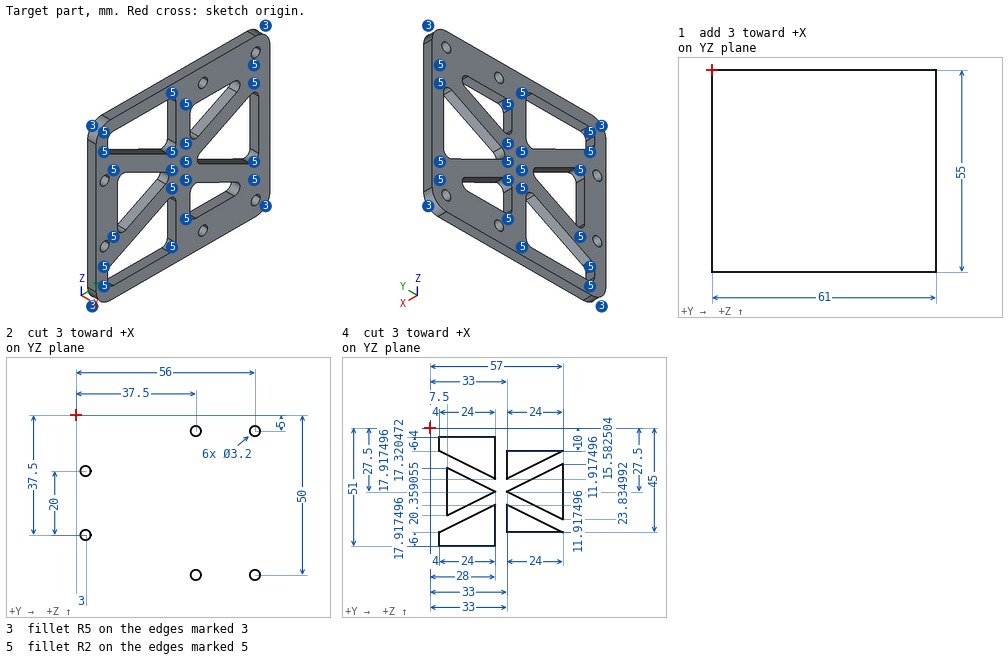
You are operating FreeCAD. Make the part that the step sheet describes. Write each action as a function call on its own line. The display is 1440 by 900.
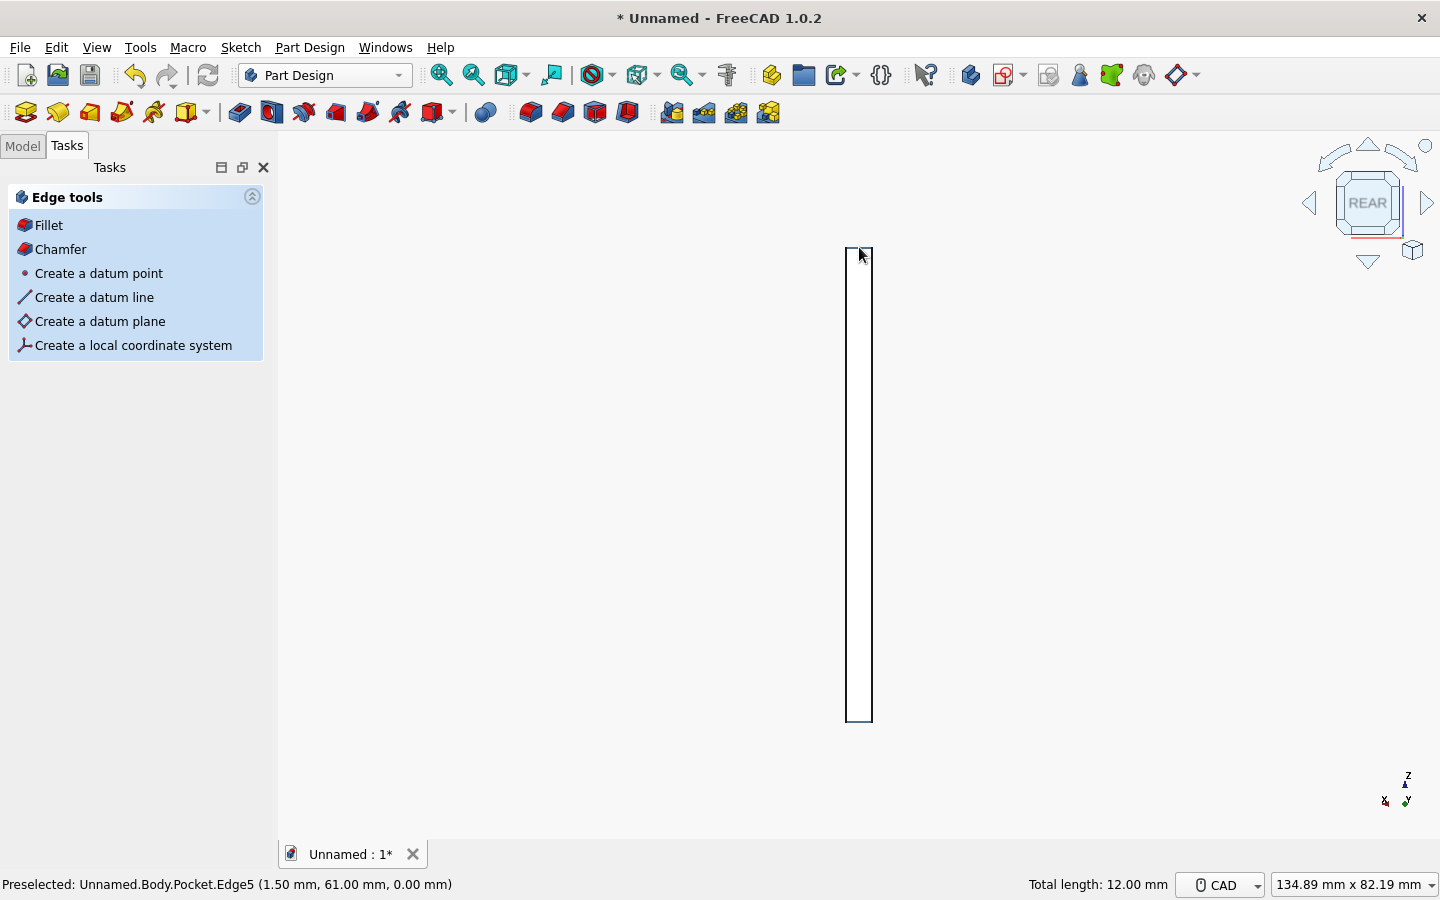
click(532, 112)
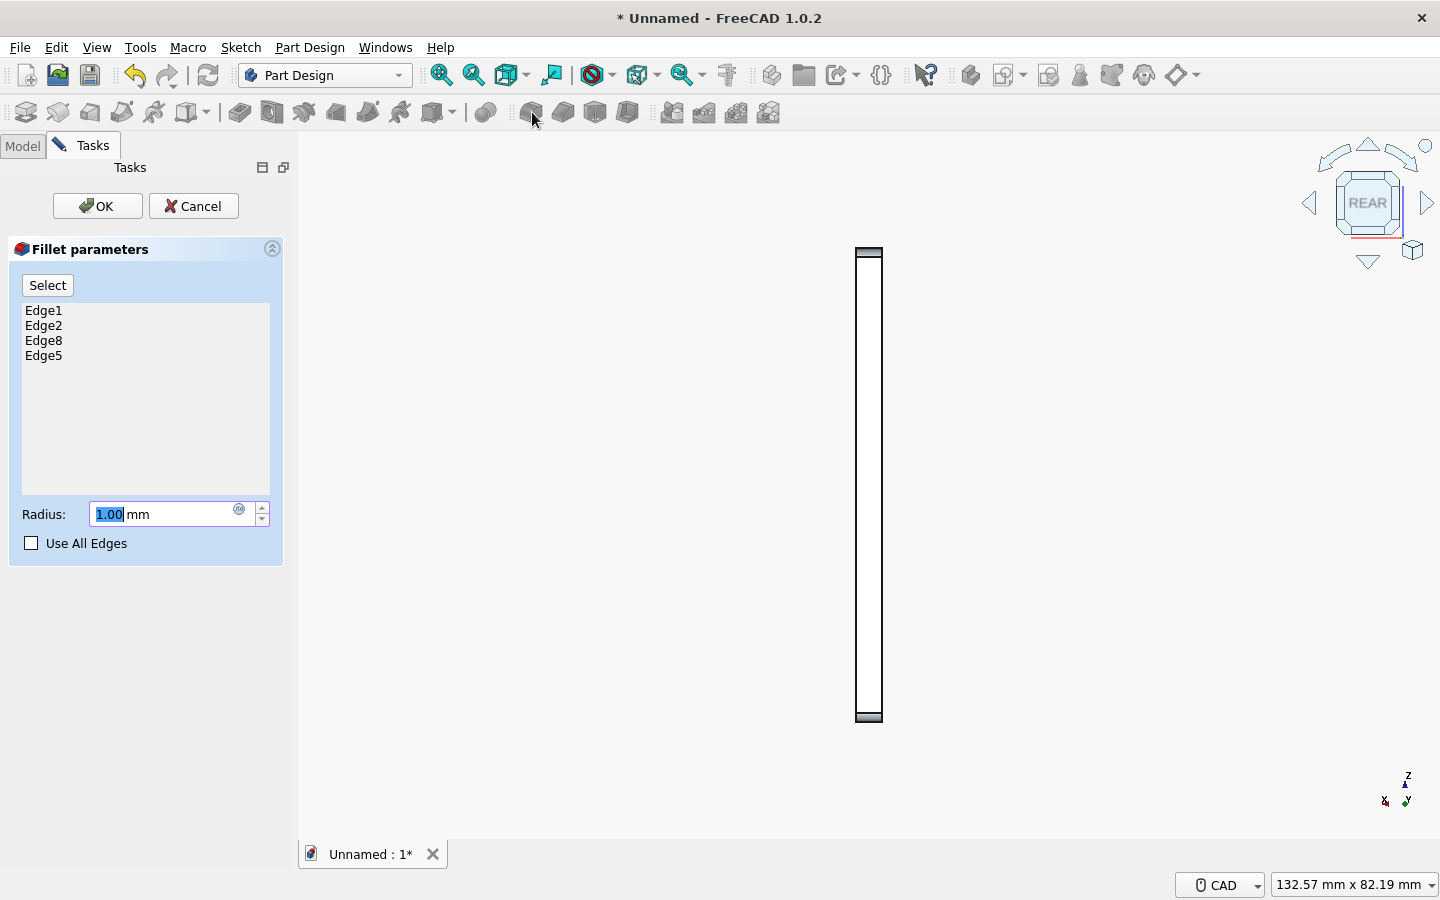
text(5)
key(Tab)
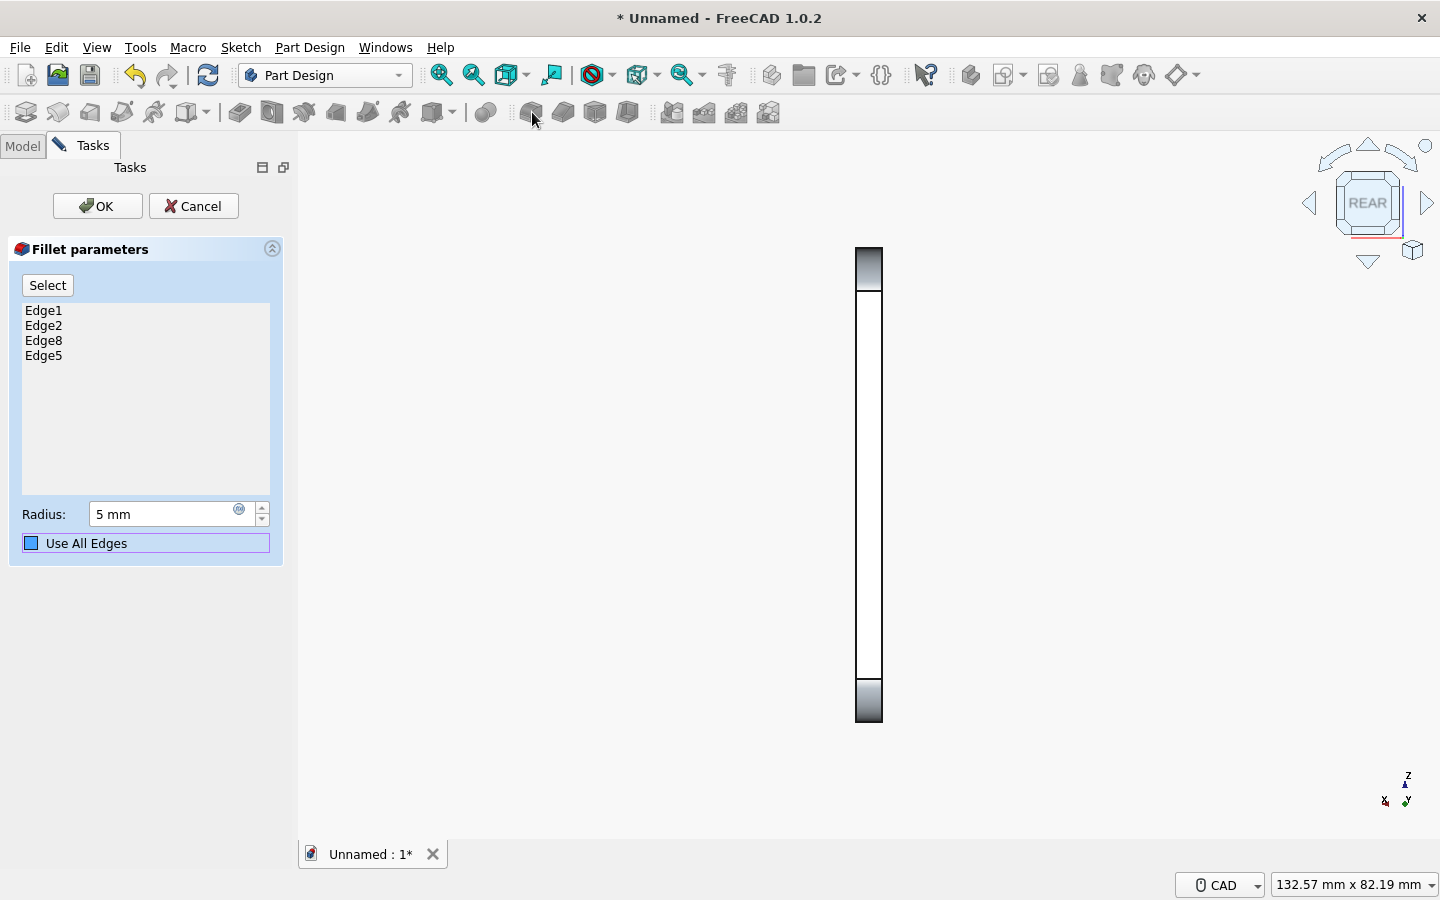
click(98, 206)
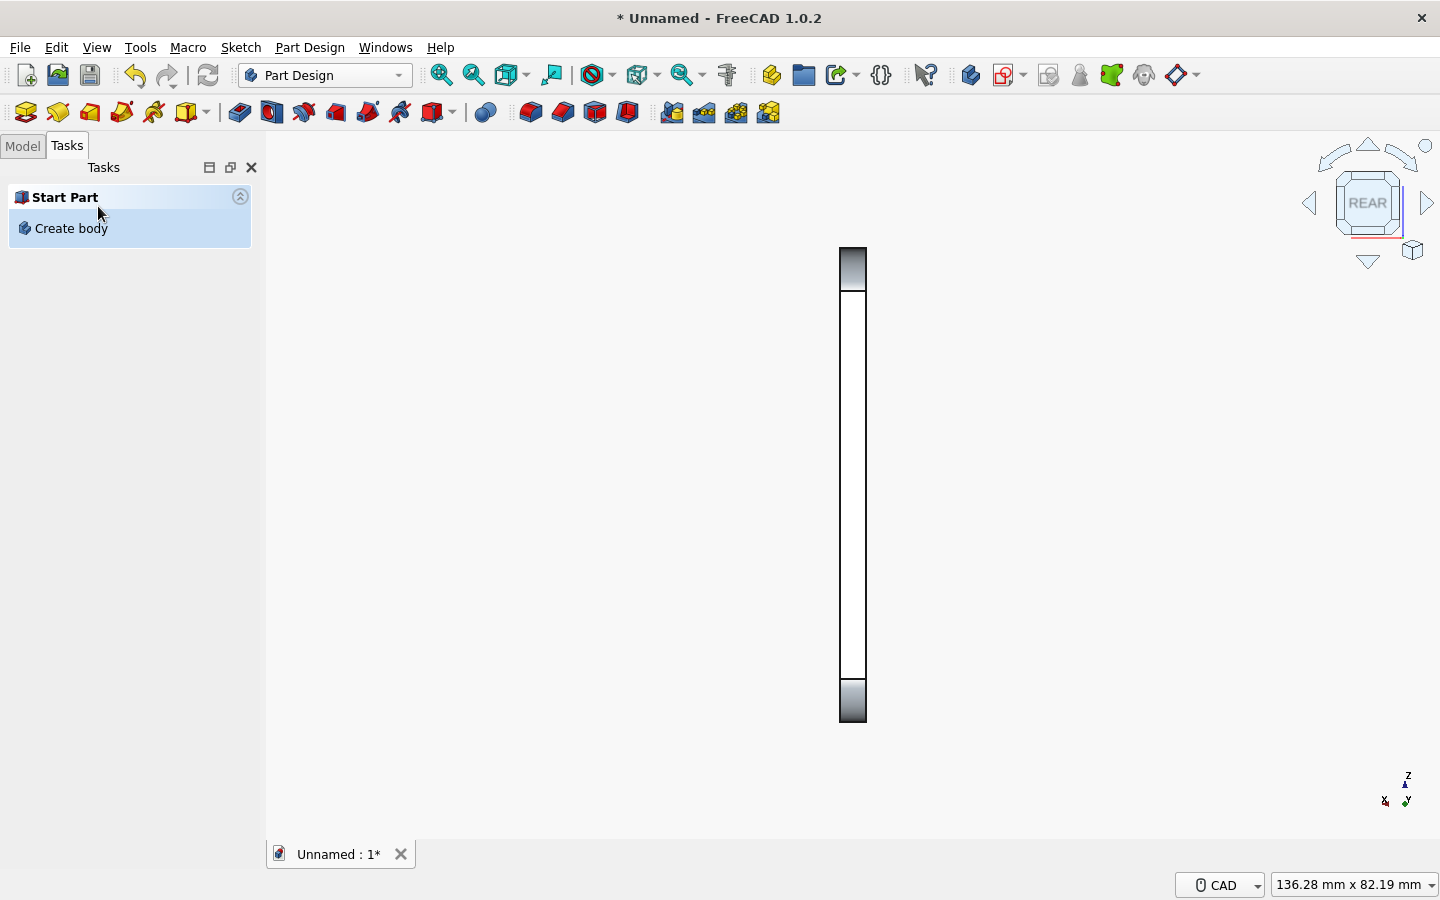
click(1004, 76)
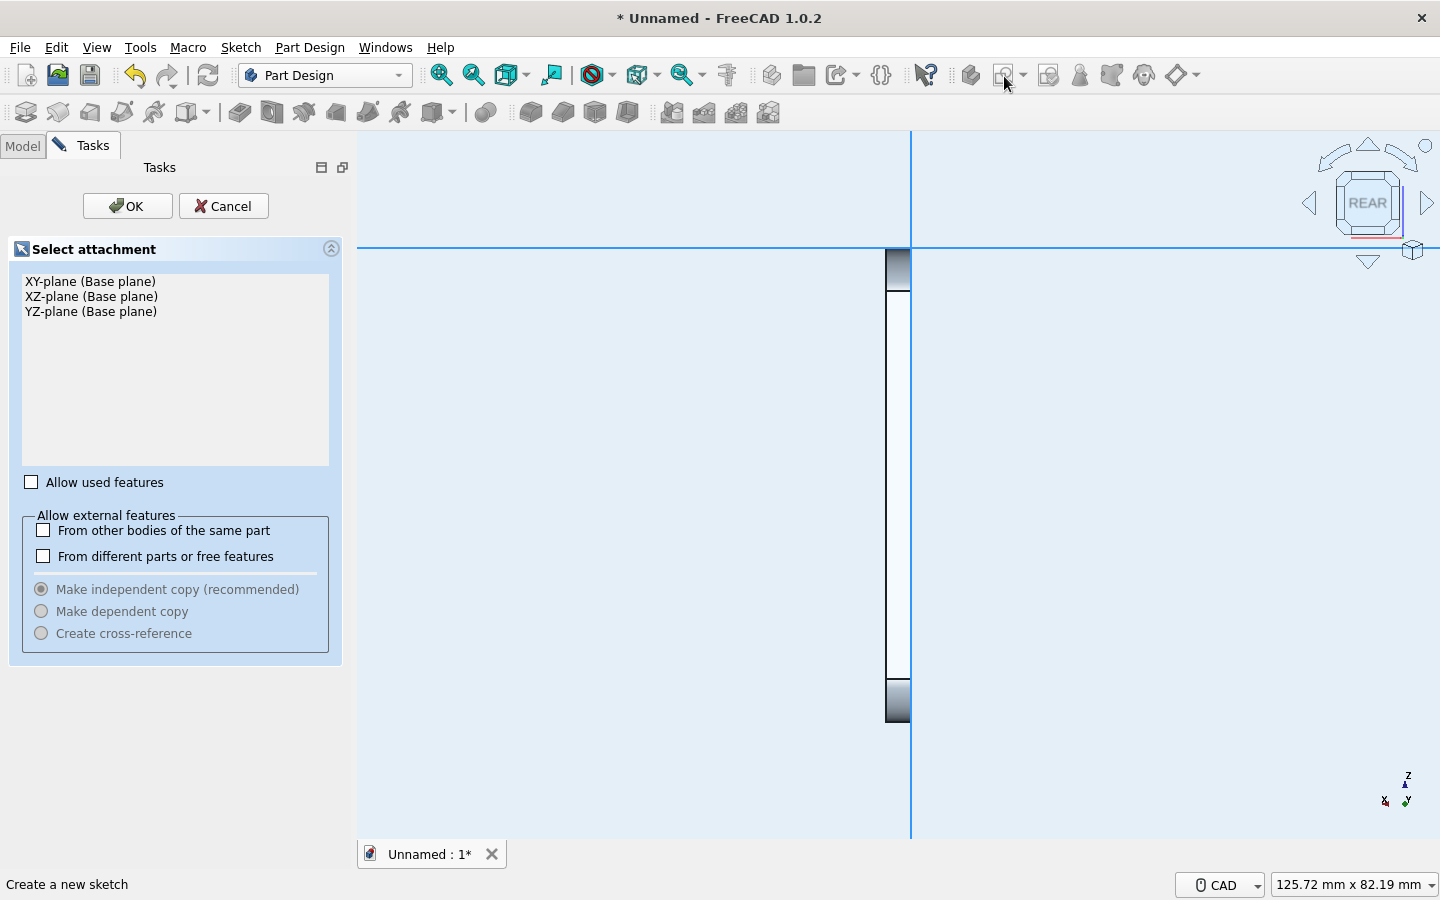
click(82, 312)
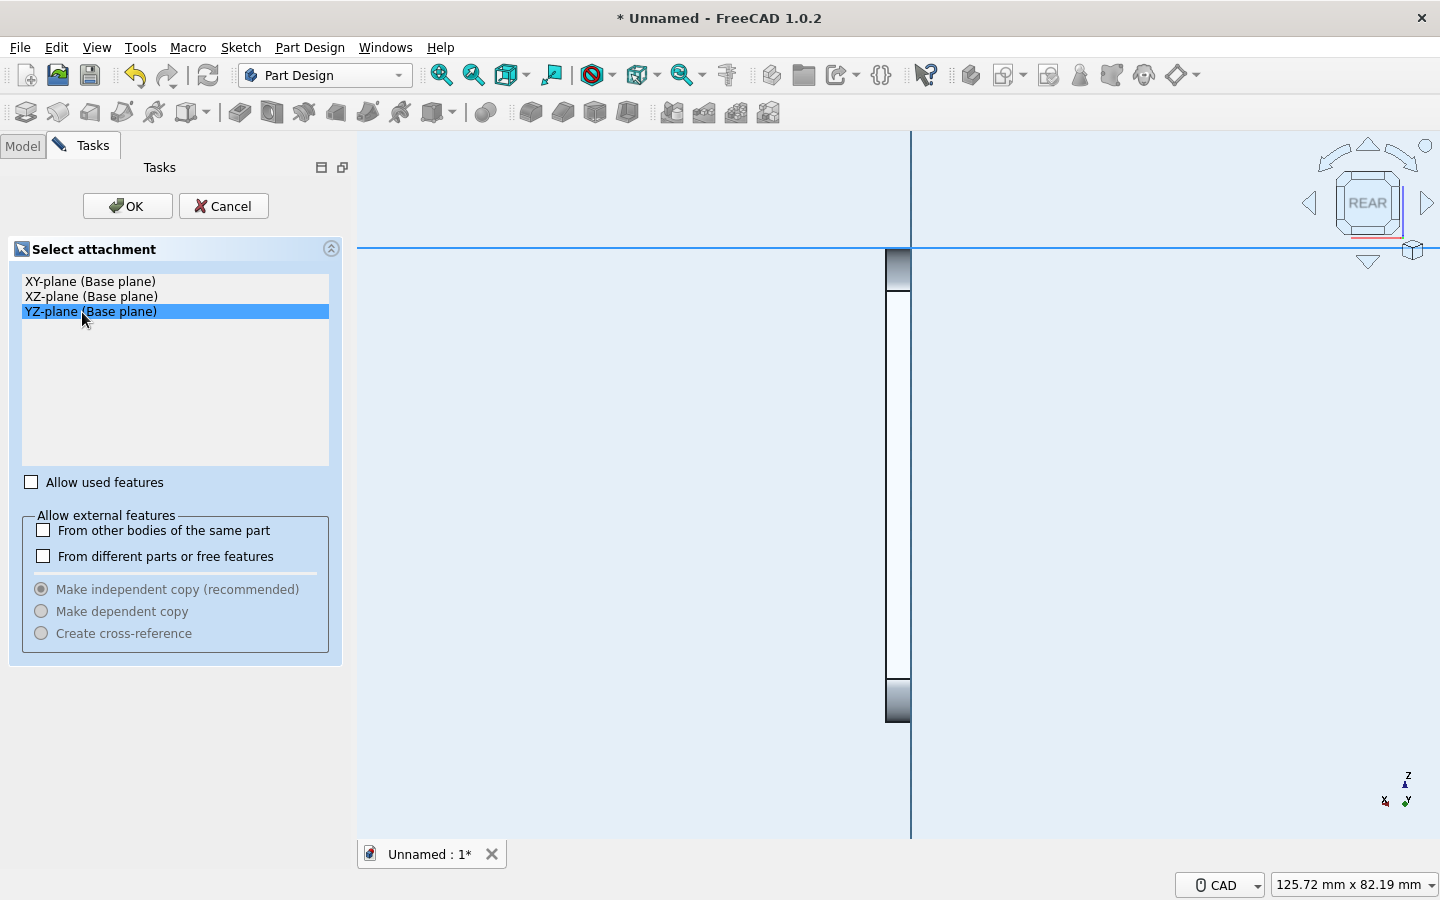
click(128, 206)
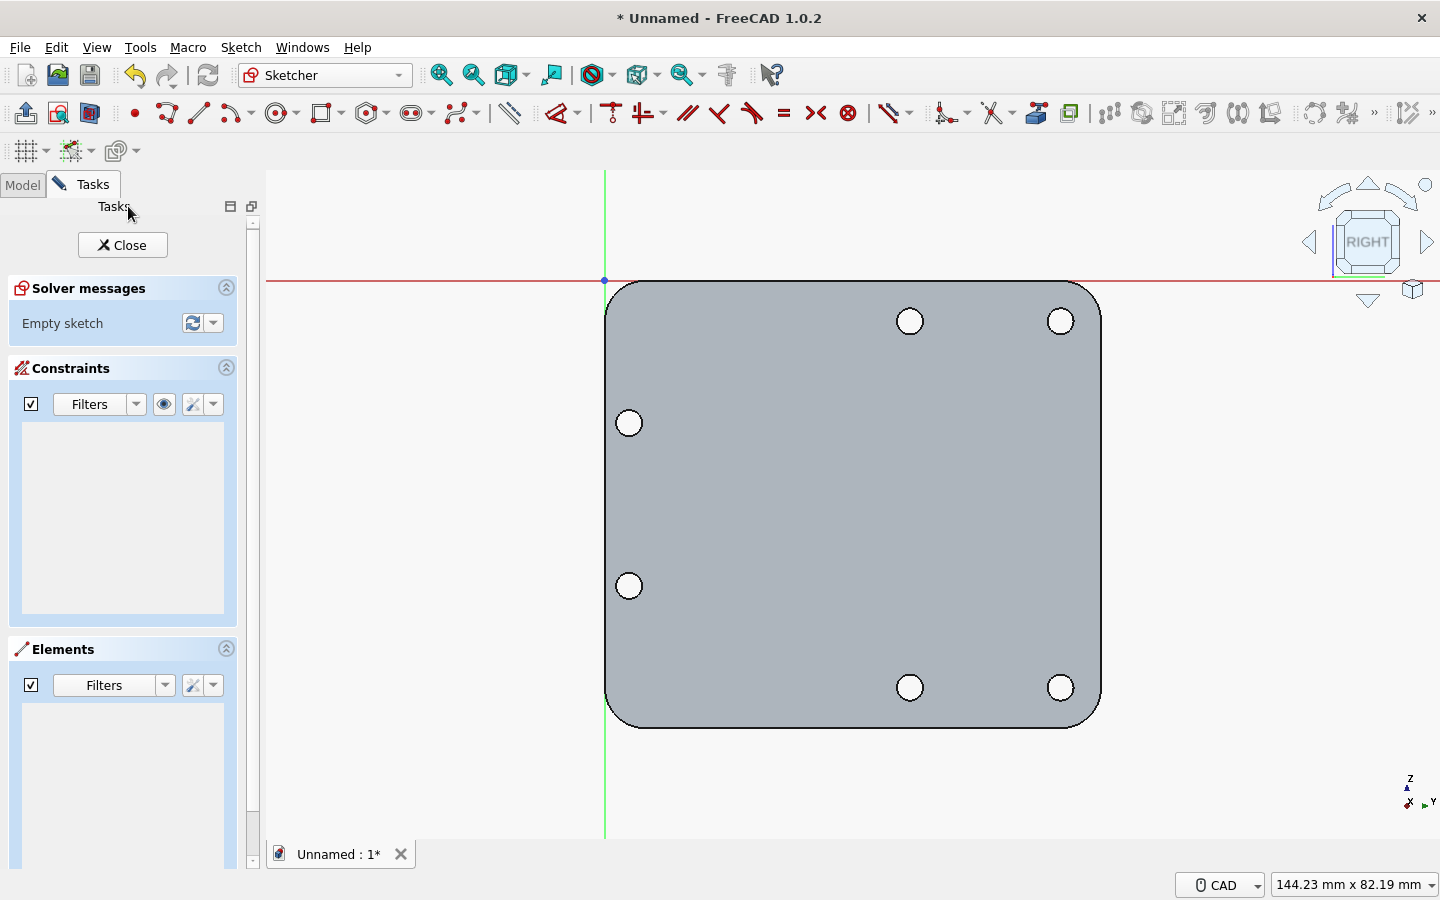
click(90, 114)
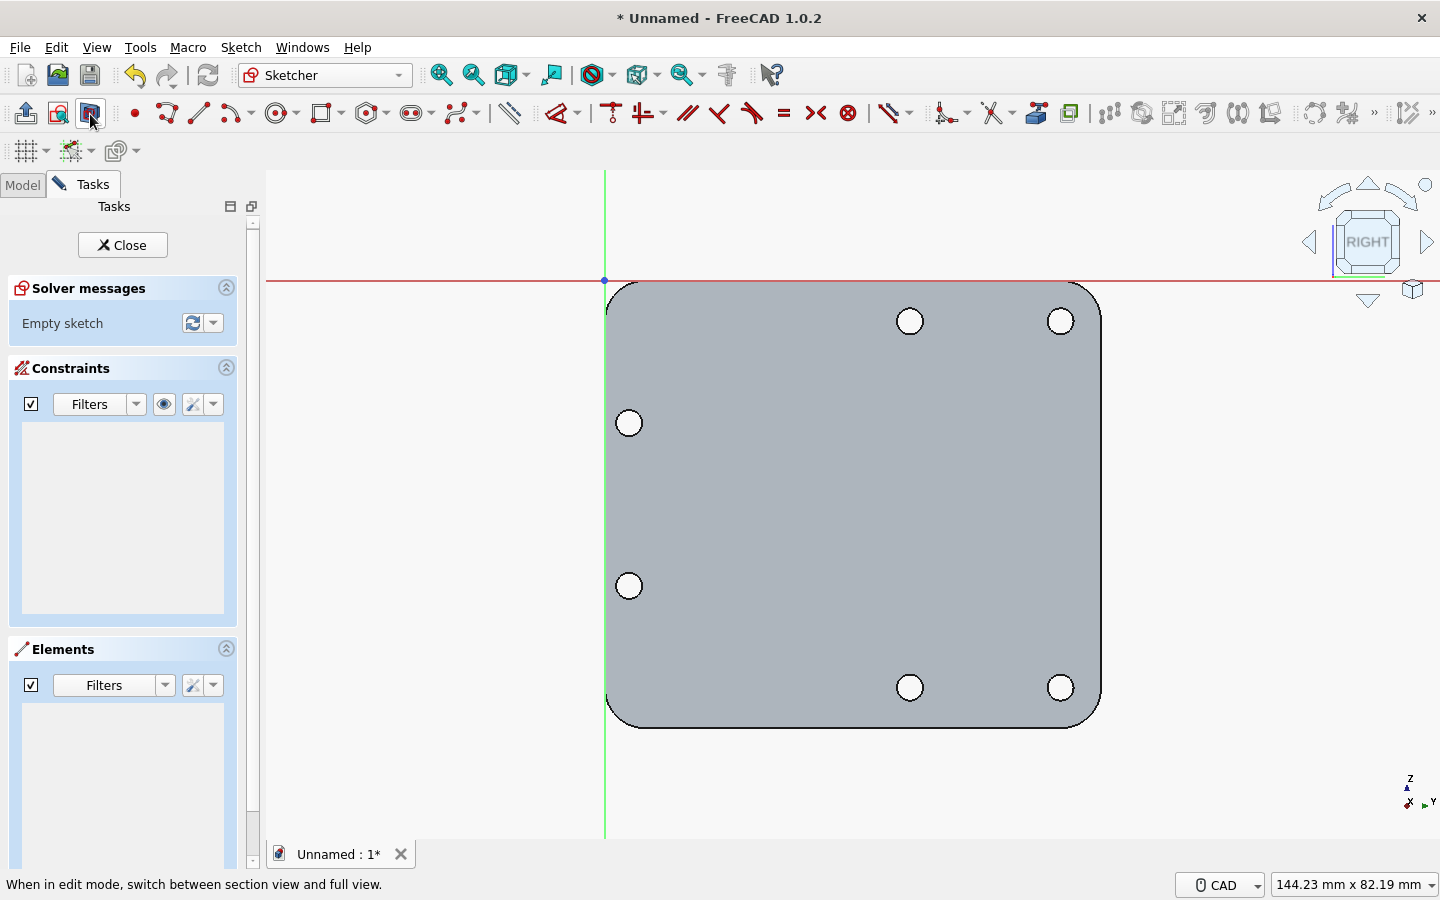
click(168, 114)